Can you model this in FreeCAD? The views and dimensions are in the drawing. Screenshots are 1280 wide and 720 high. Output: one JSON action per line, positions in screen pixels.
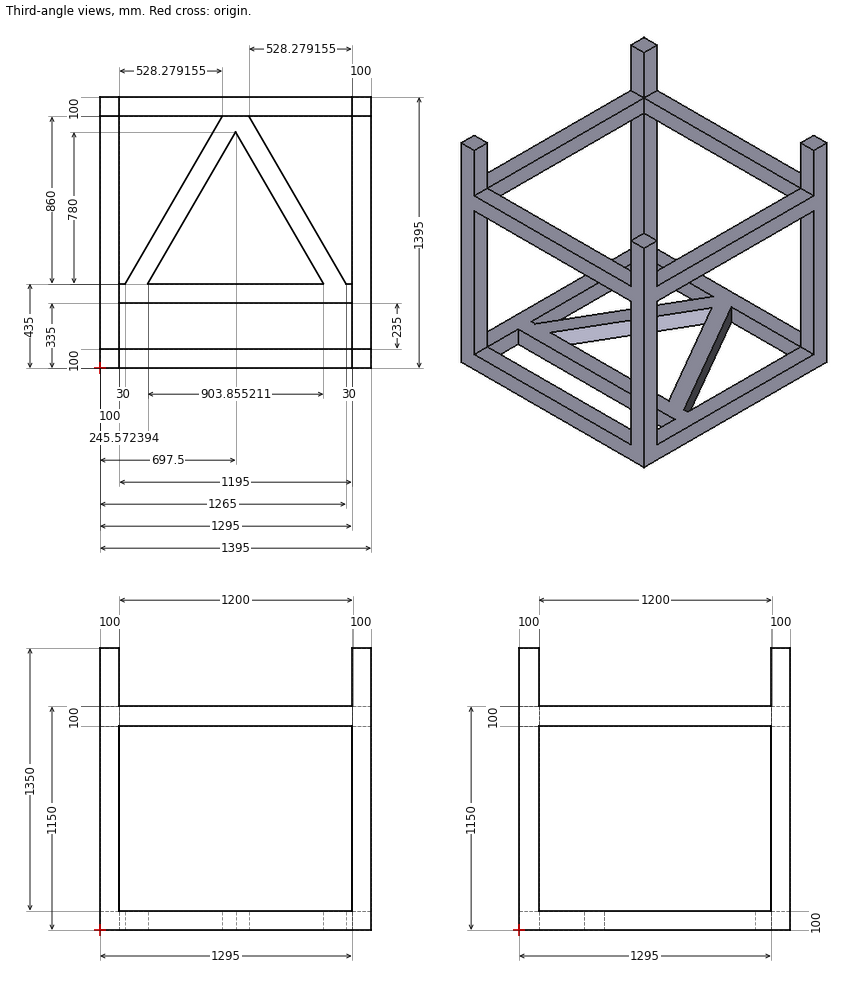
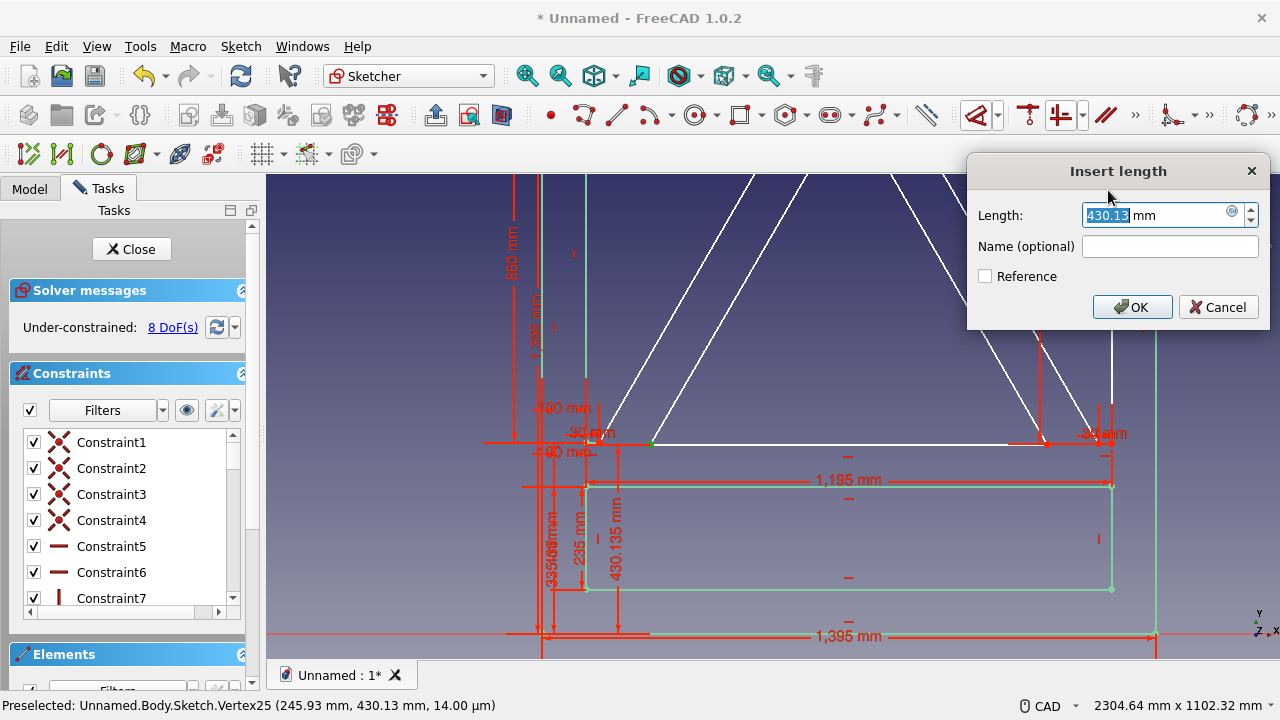
{"action": "type", "text": "435"}
{"action": "key", "text": "Return"}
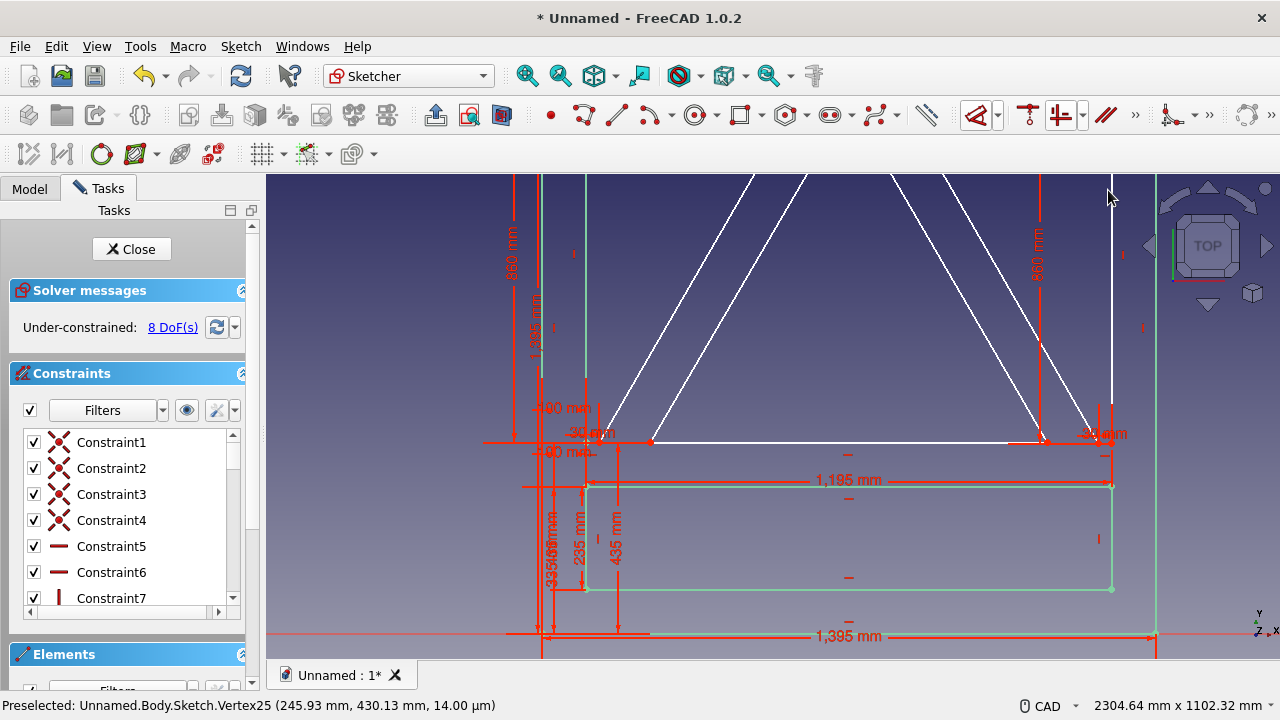
{"action": "left_click", "coordinate": [1099, 444]}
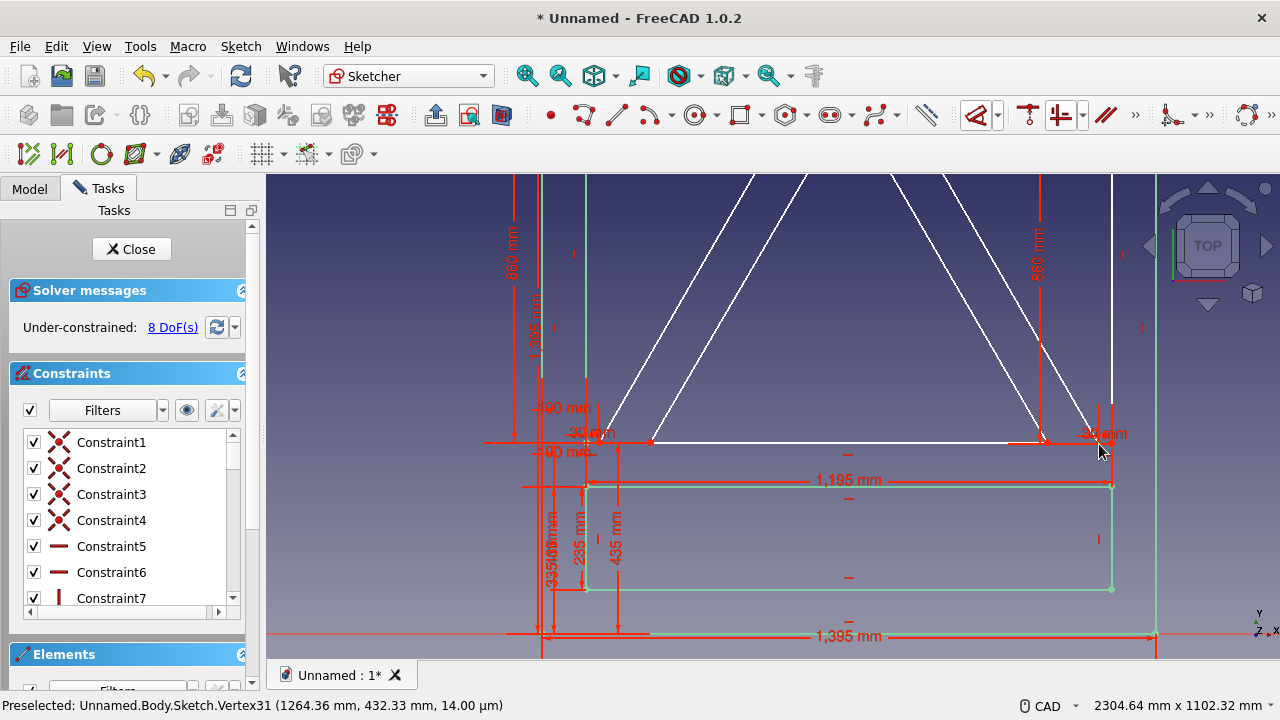
{"action": "left_click", "coordinate": [998, 116]}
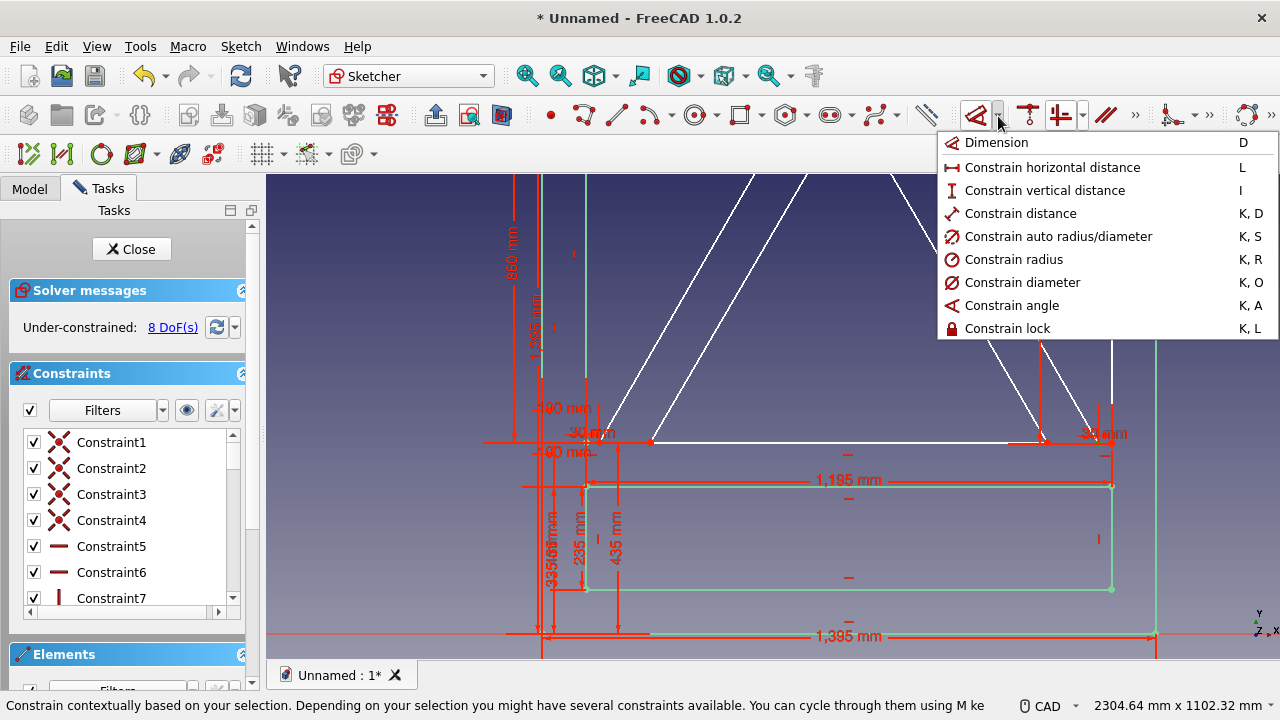
{"action": "left_click", "coordinate": [1108, 190]}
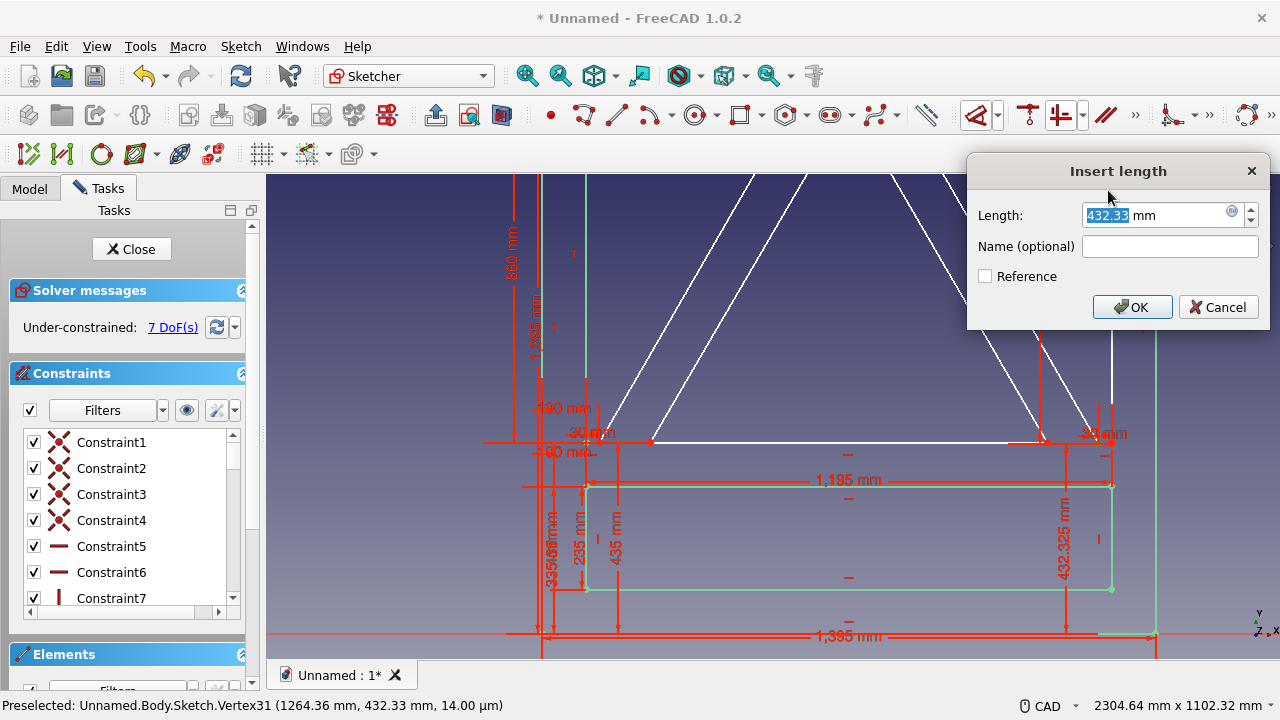
{"action": "type", "text": "435"}
{"action": "key", "text": "Return"}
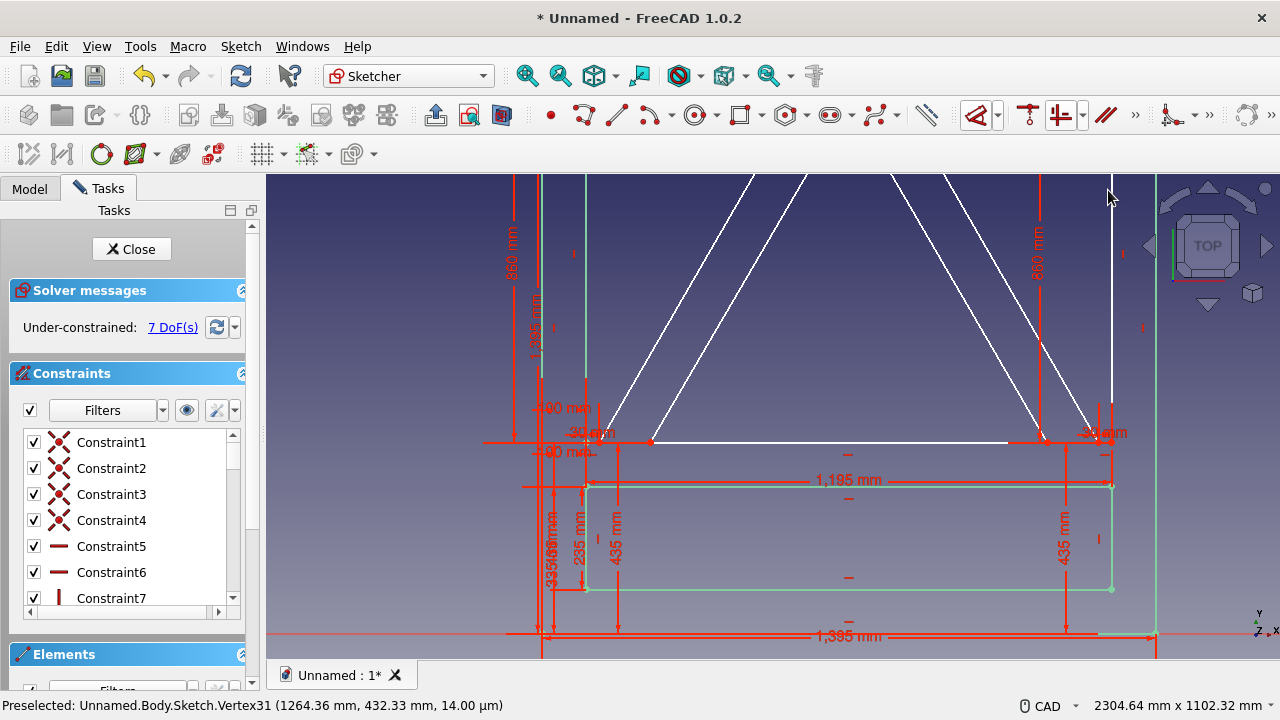
{"action": "left_click", "coordinate": [710, 340]}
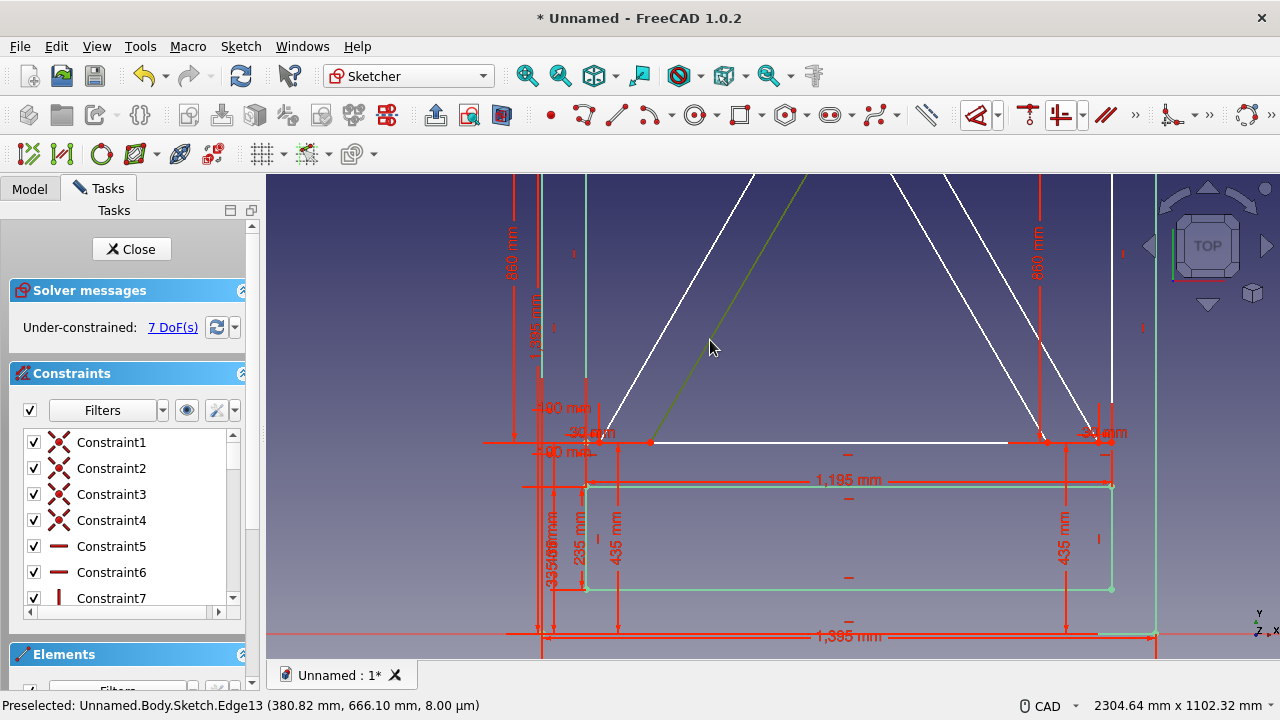
{"action": "key", "text": "i"}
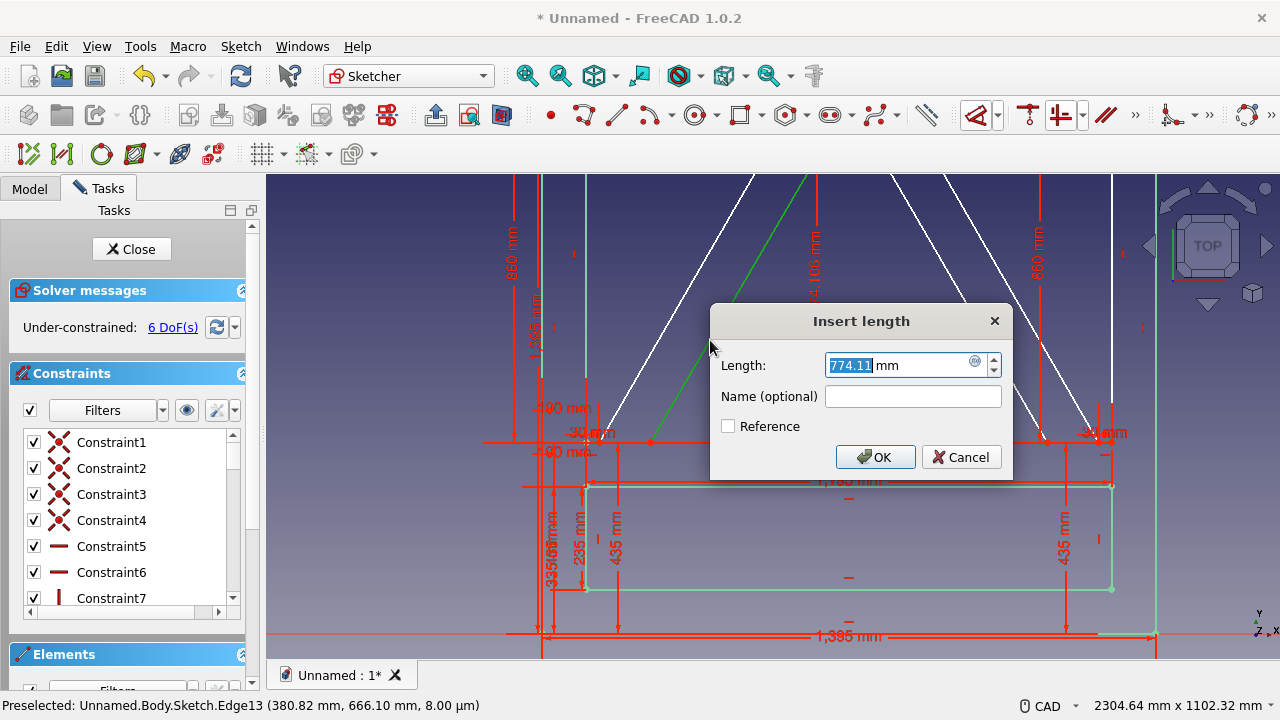
{"action": "type", "text": "780"}
{"action": "key", "text": "Return"}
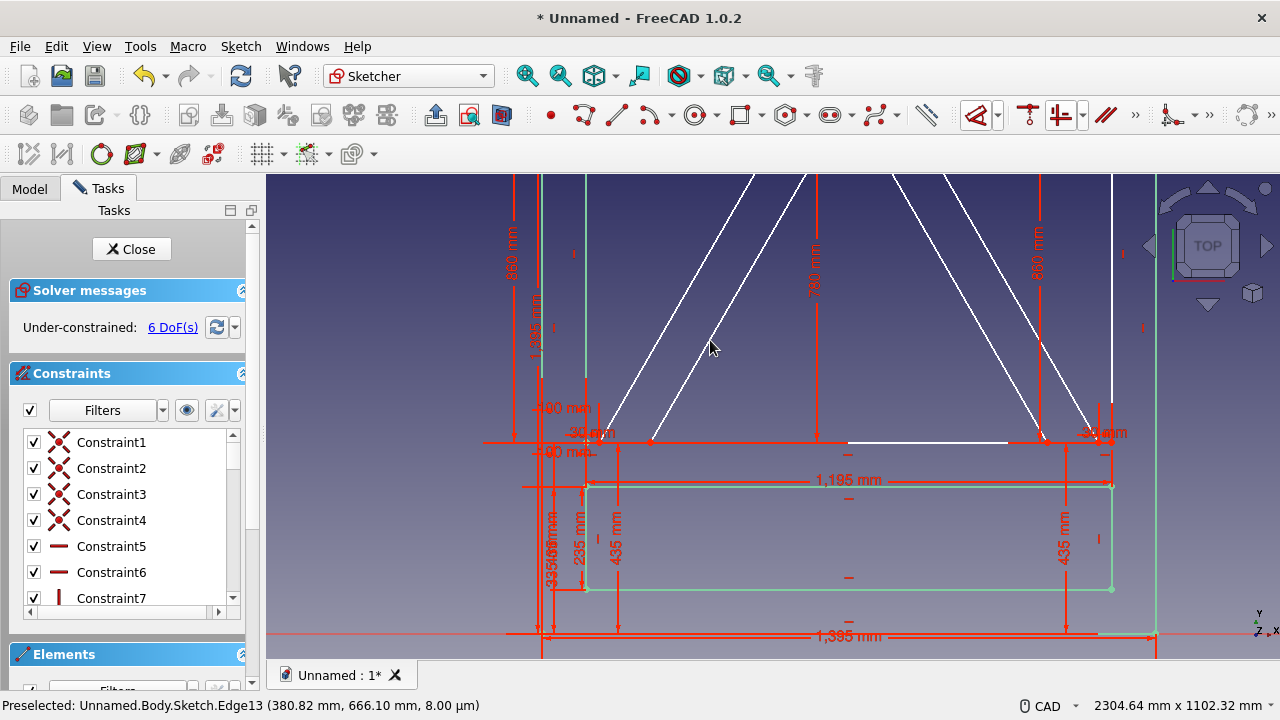
{"action": "left_click", "coordinate": [1099, 443]}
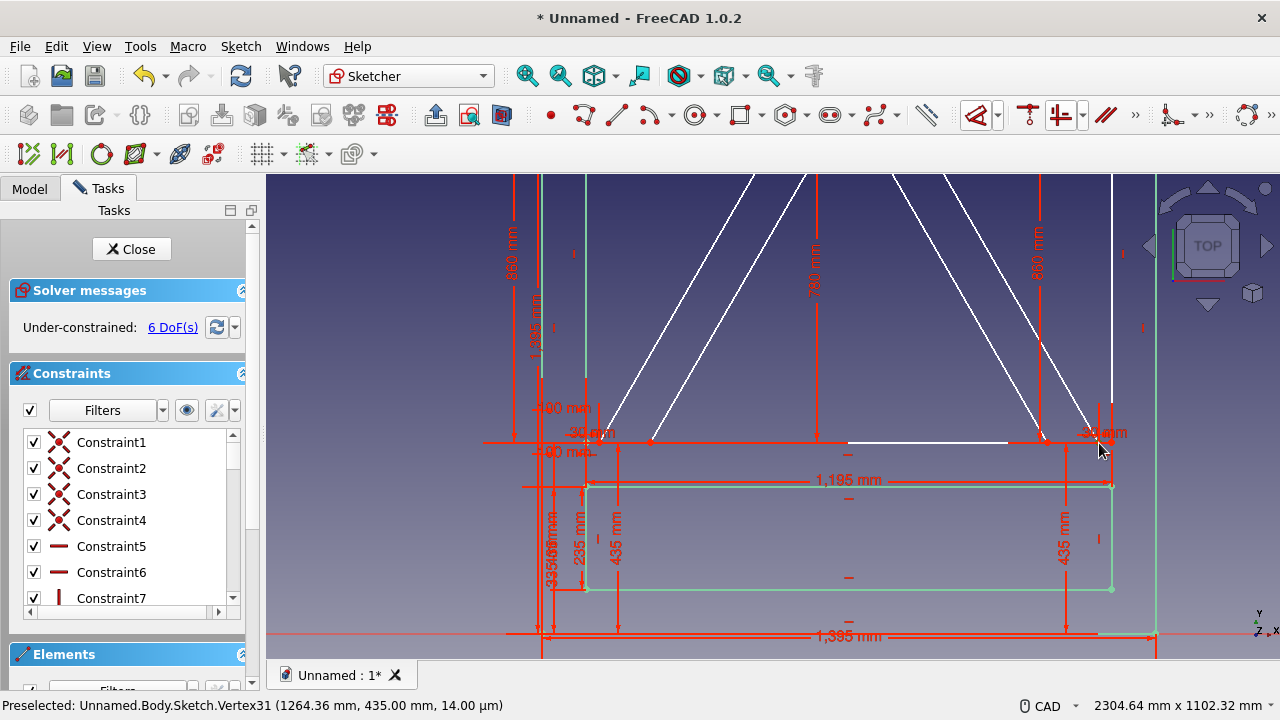
{"action": "key", "text": "l"}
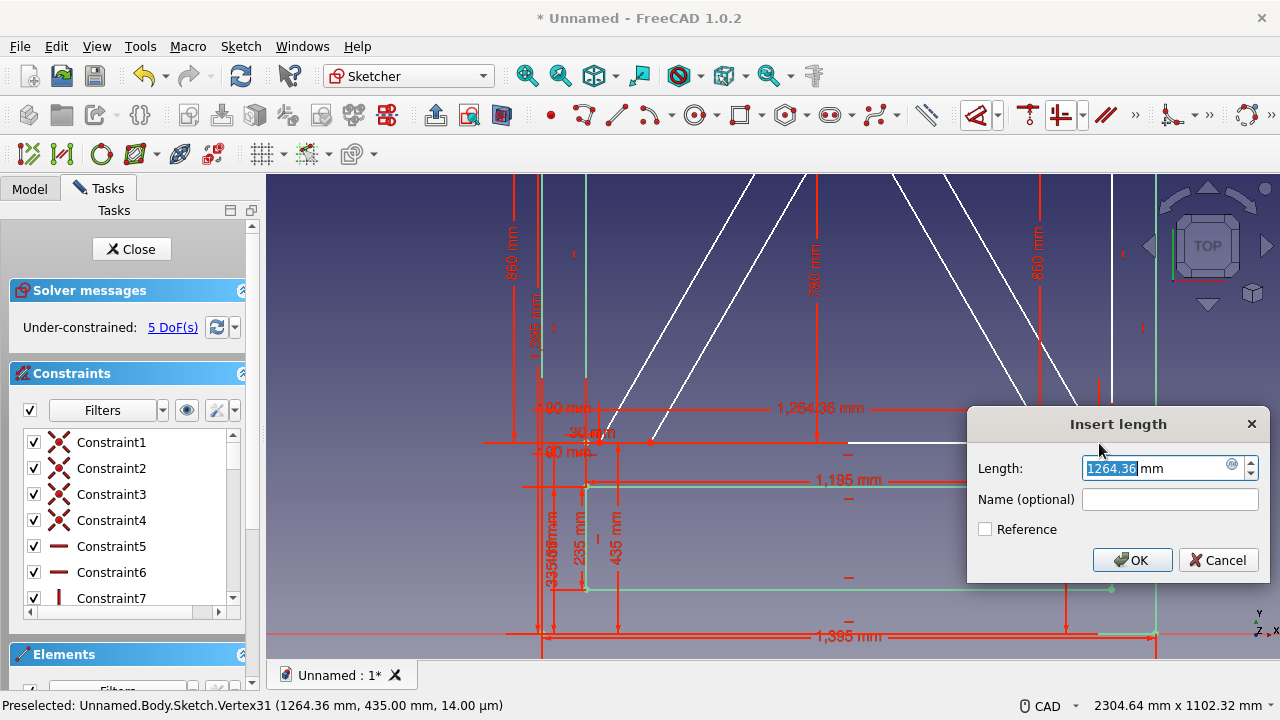
{"action": "type", "text": "1265"}
{"action": "key", "text": "Return"}